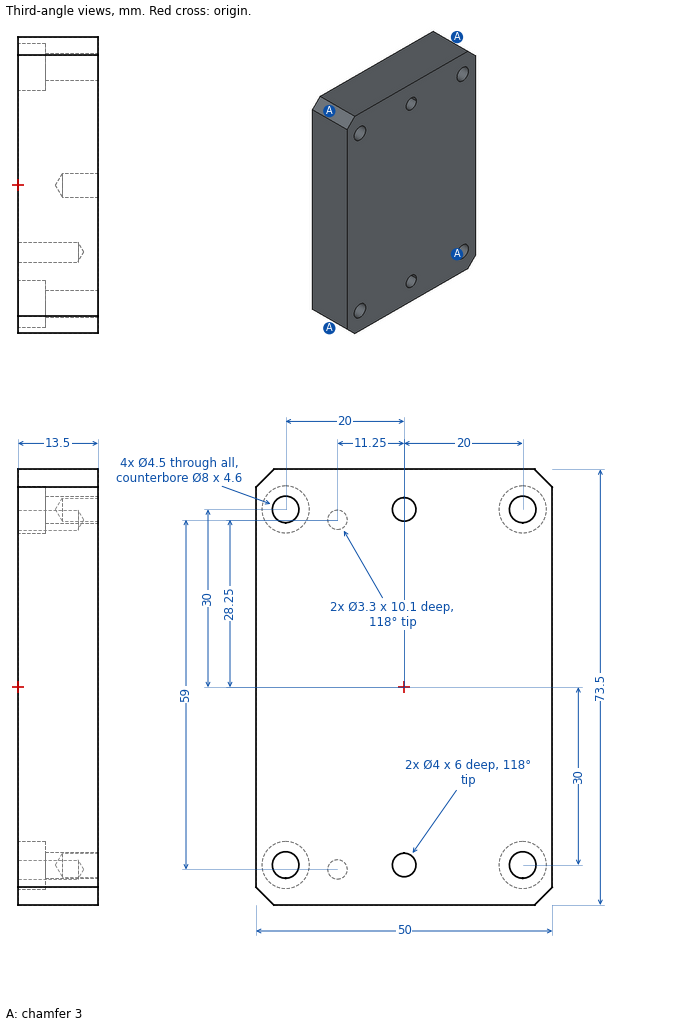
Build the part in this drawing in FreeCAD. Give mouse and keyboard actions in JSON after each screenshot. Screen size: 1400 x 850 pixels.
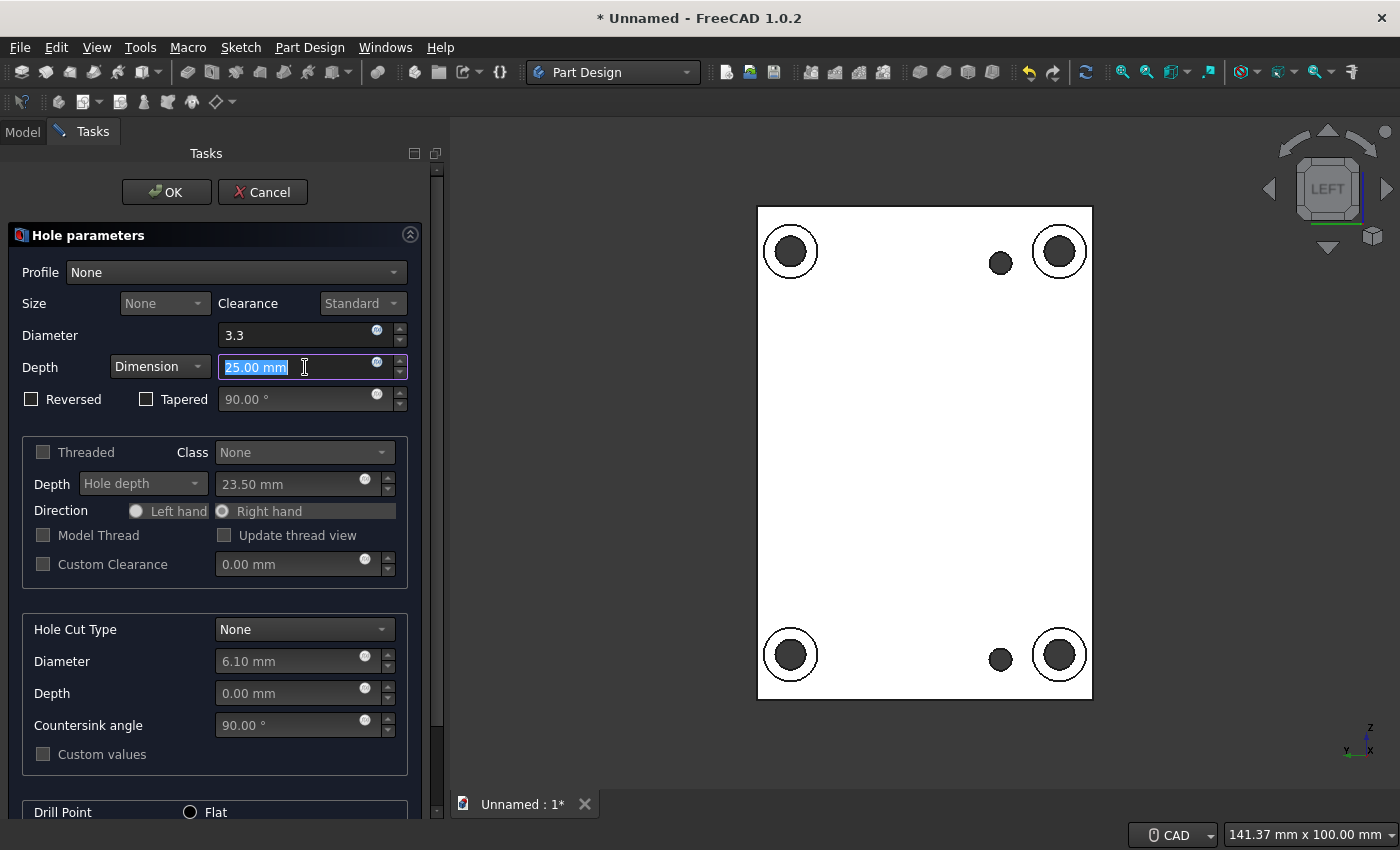
{"action": "type", "text": "10.1"}
{"action": "key", "text": "Tab"}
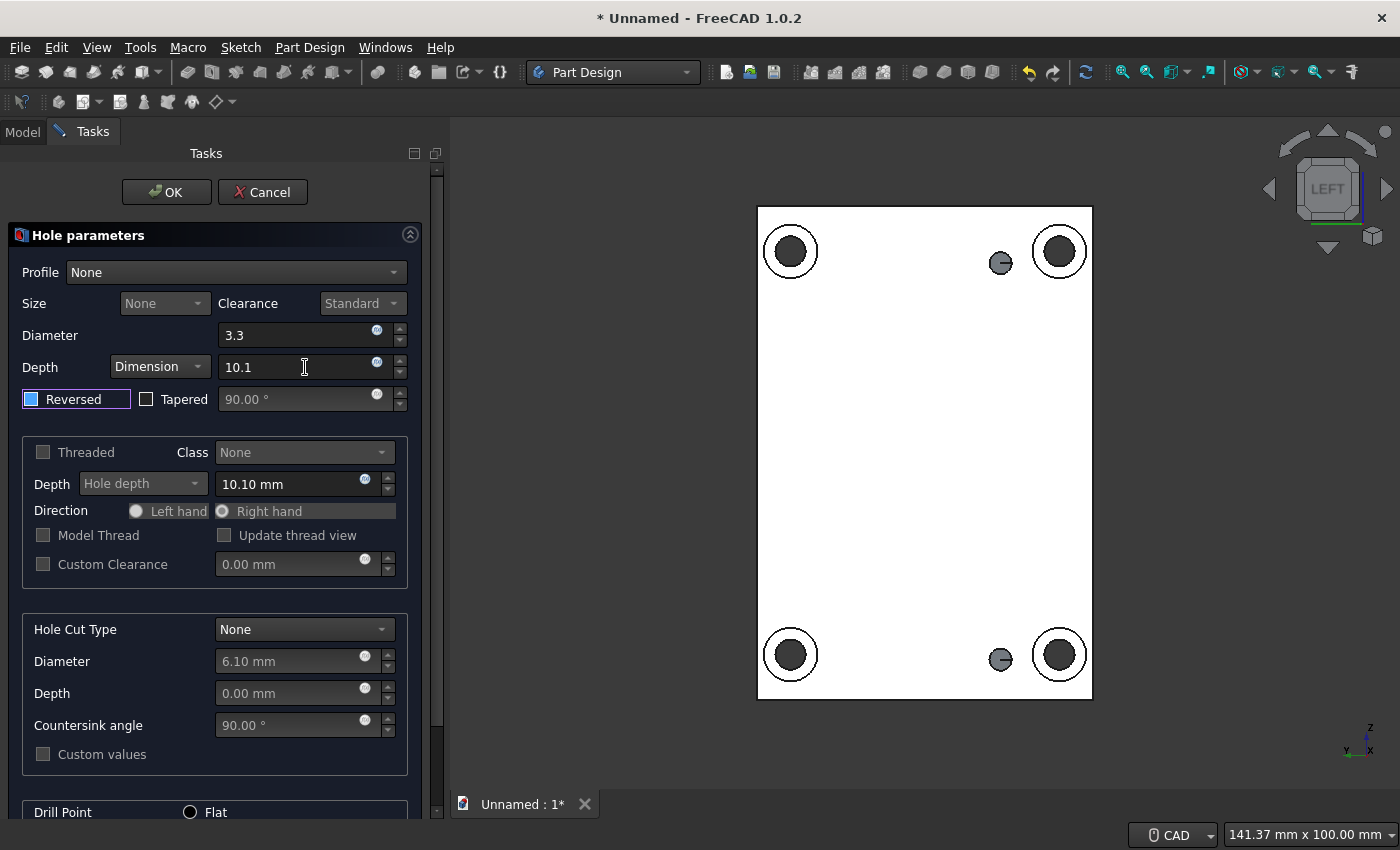
{"action": "left_click", "coordinate": [167, 192]}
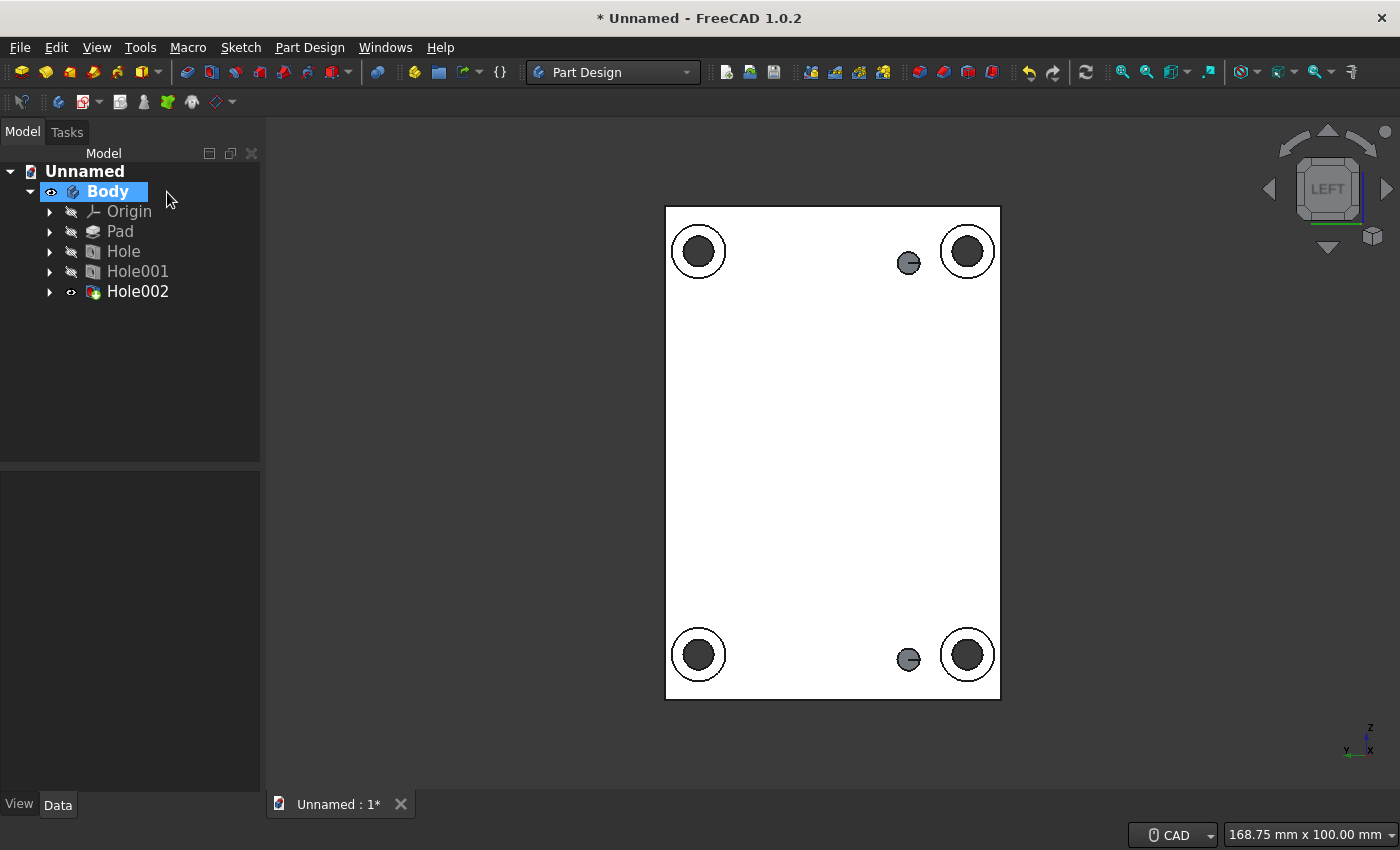
{"action": "key", "text": "0"}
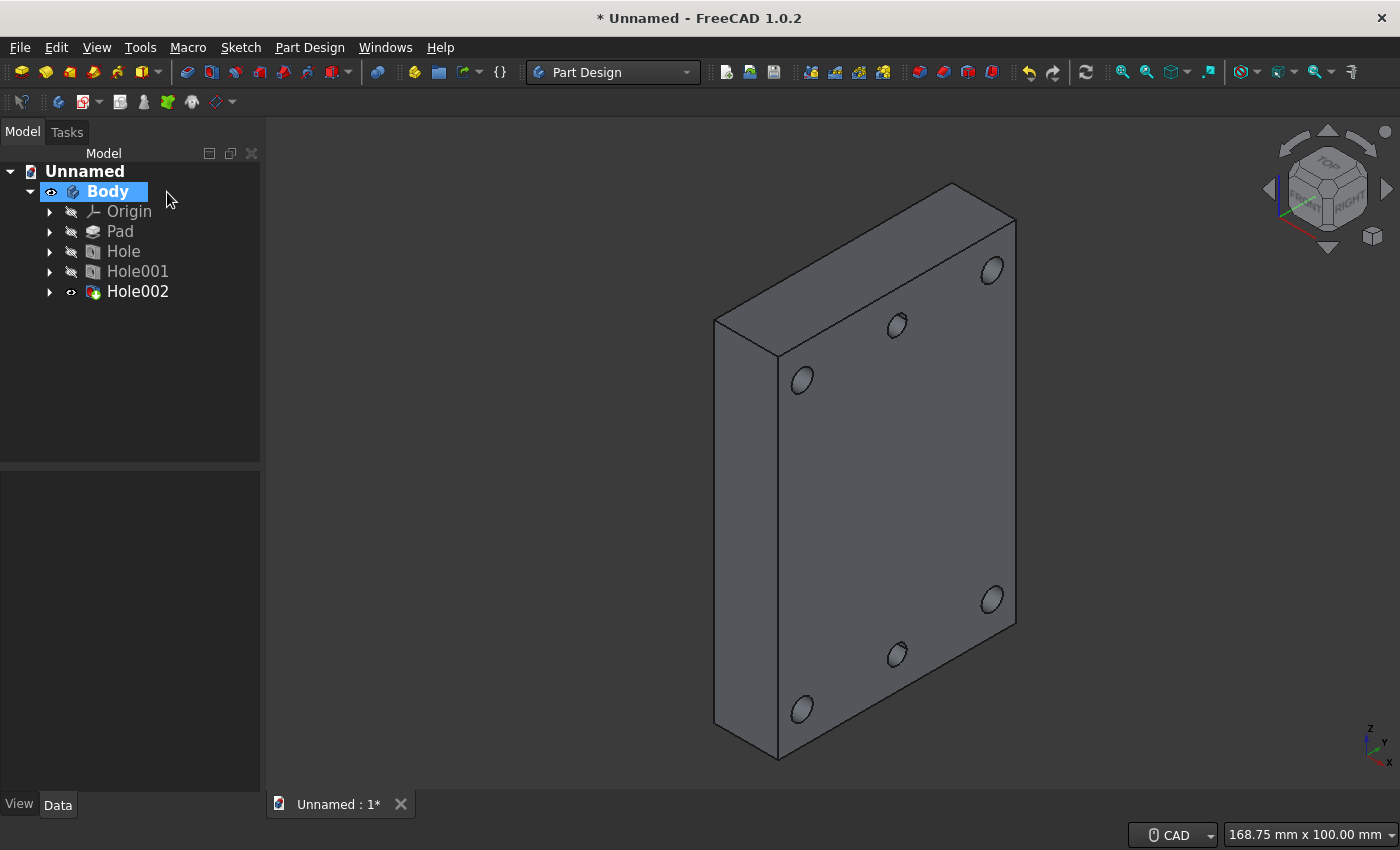
{"action": "left_click", "coordinate": [746, 337]}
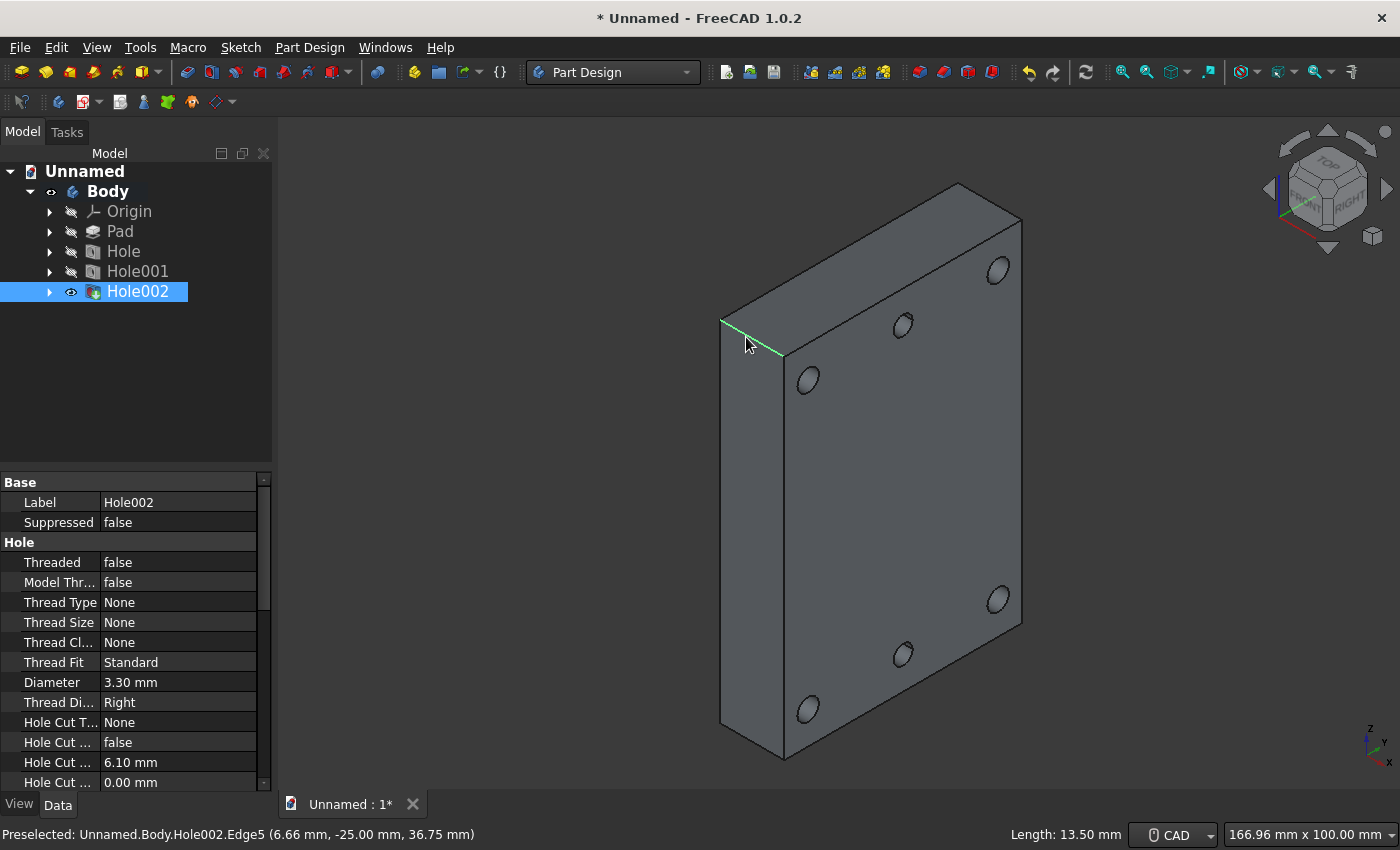
{"action": "key", "text": "2"}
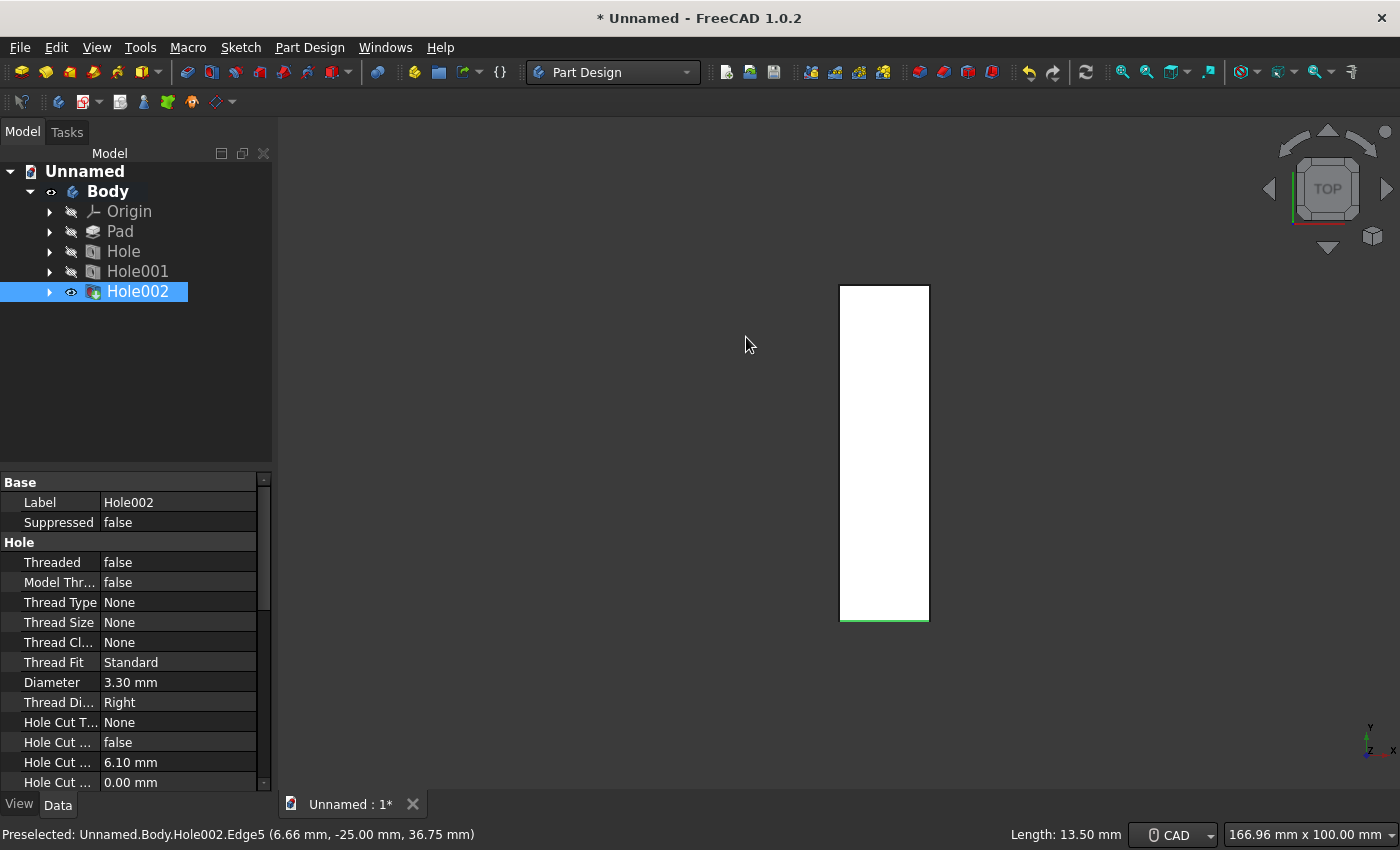
{"action": "left_click", "coordinate": [884, 284], "text": "ctrl"}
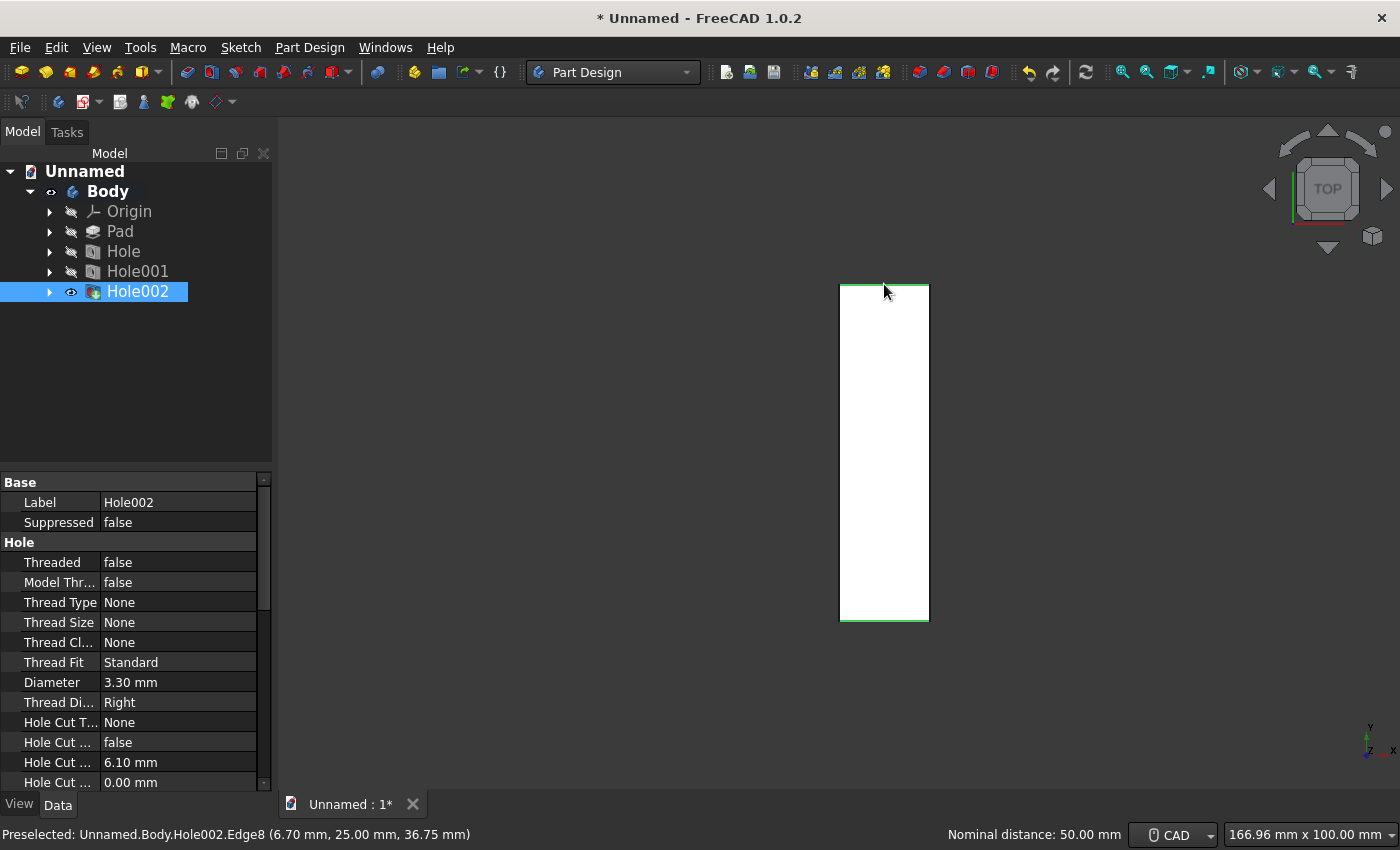
{"action": "key", "text": "1"}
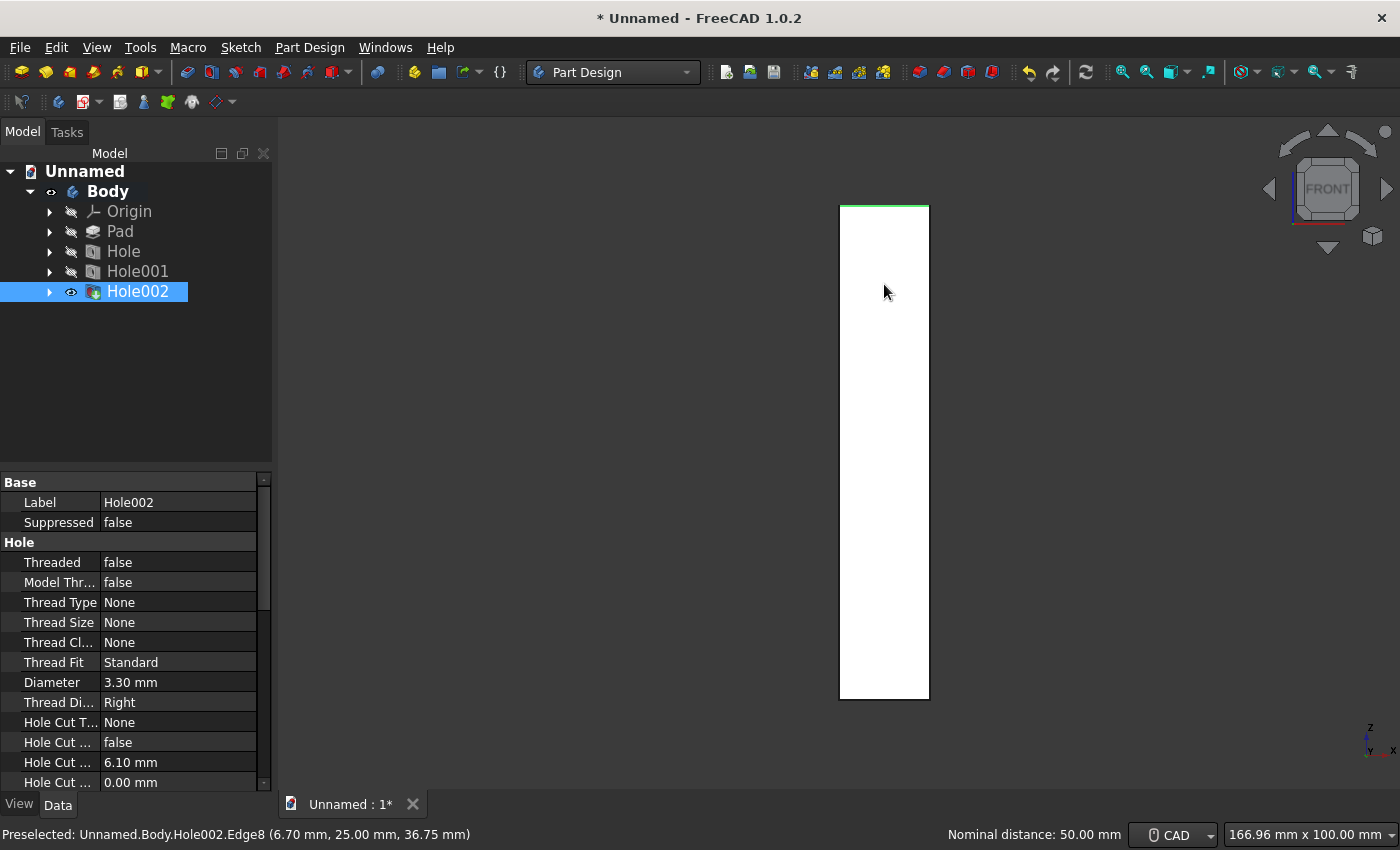
{"action": "left_click", "coordinate": [884, 699], "text": "ctrl"}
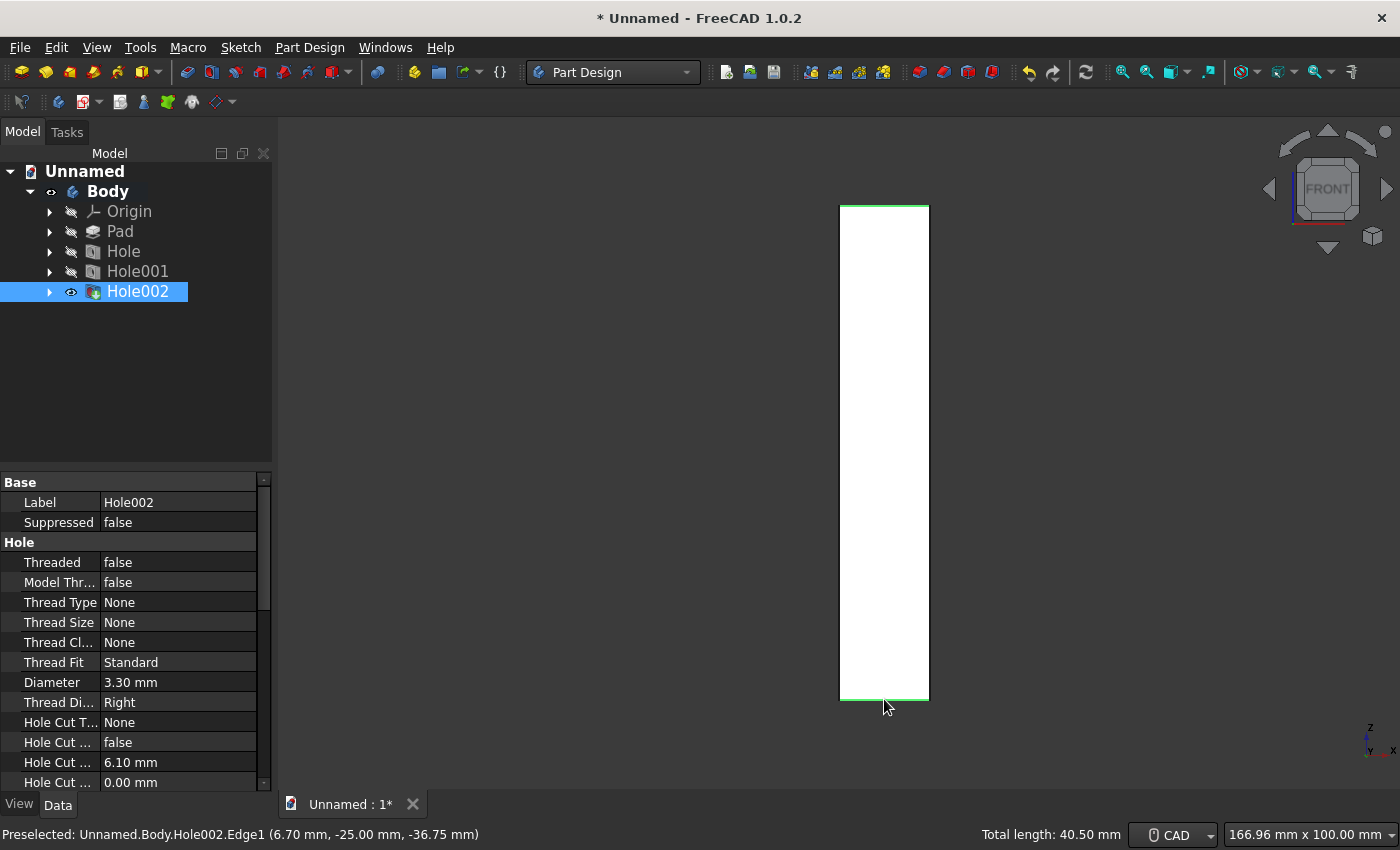
{"action": "key", "text": "3"}